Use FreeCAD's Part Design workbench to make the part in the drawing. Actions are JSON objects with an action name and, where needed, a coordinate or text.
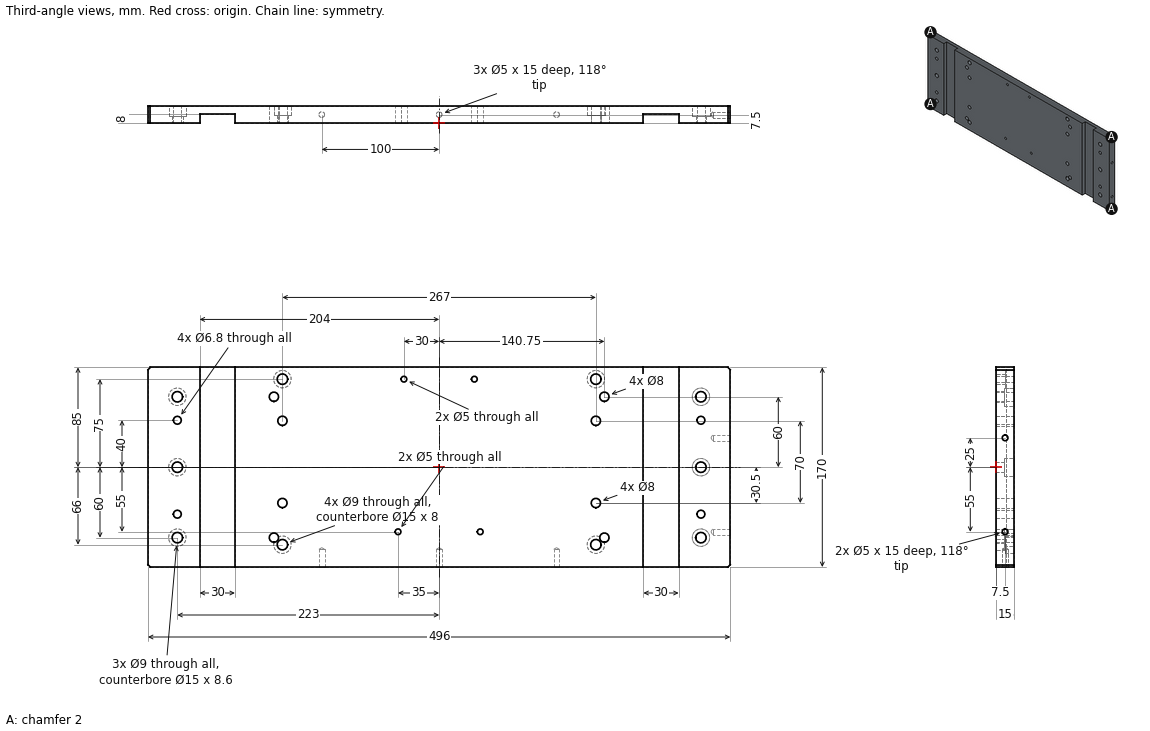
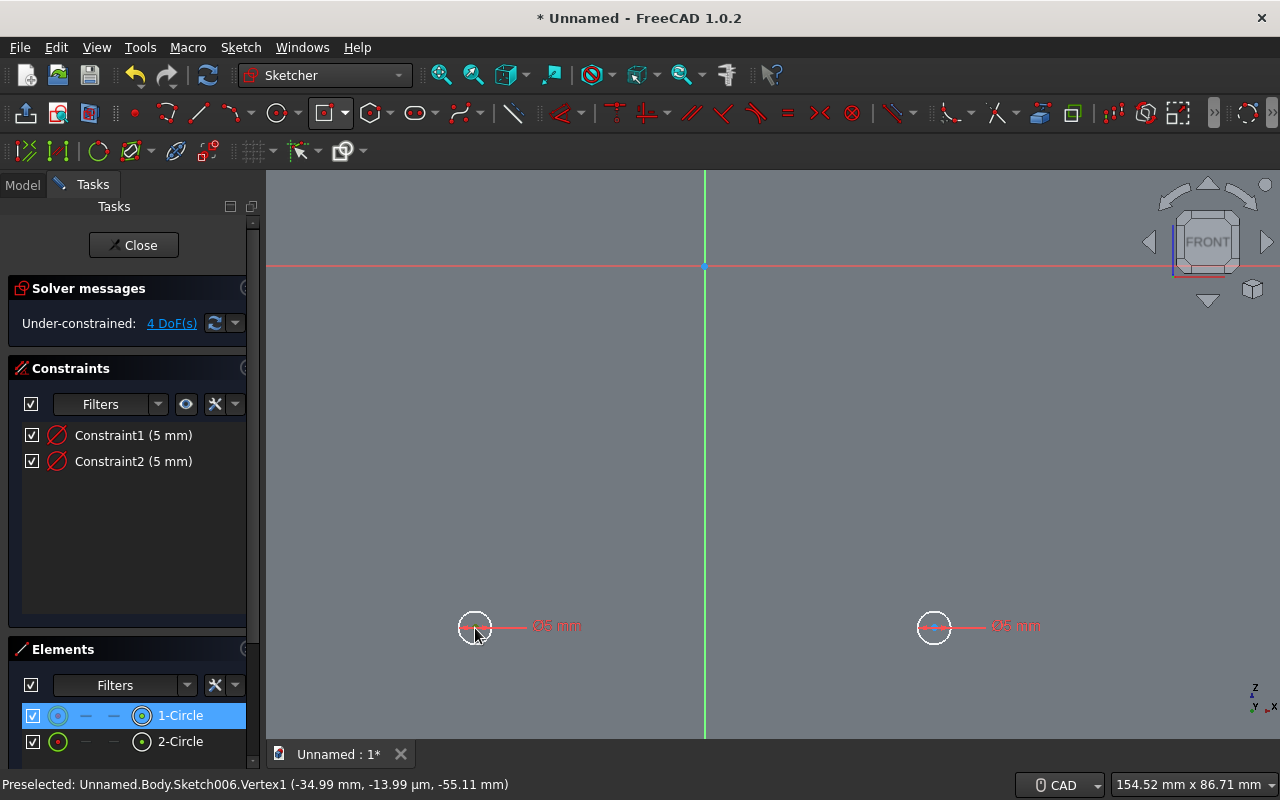
{"action": "left_click", "coordinate": [934, 628]}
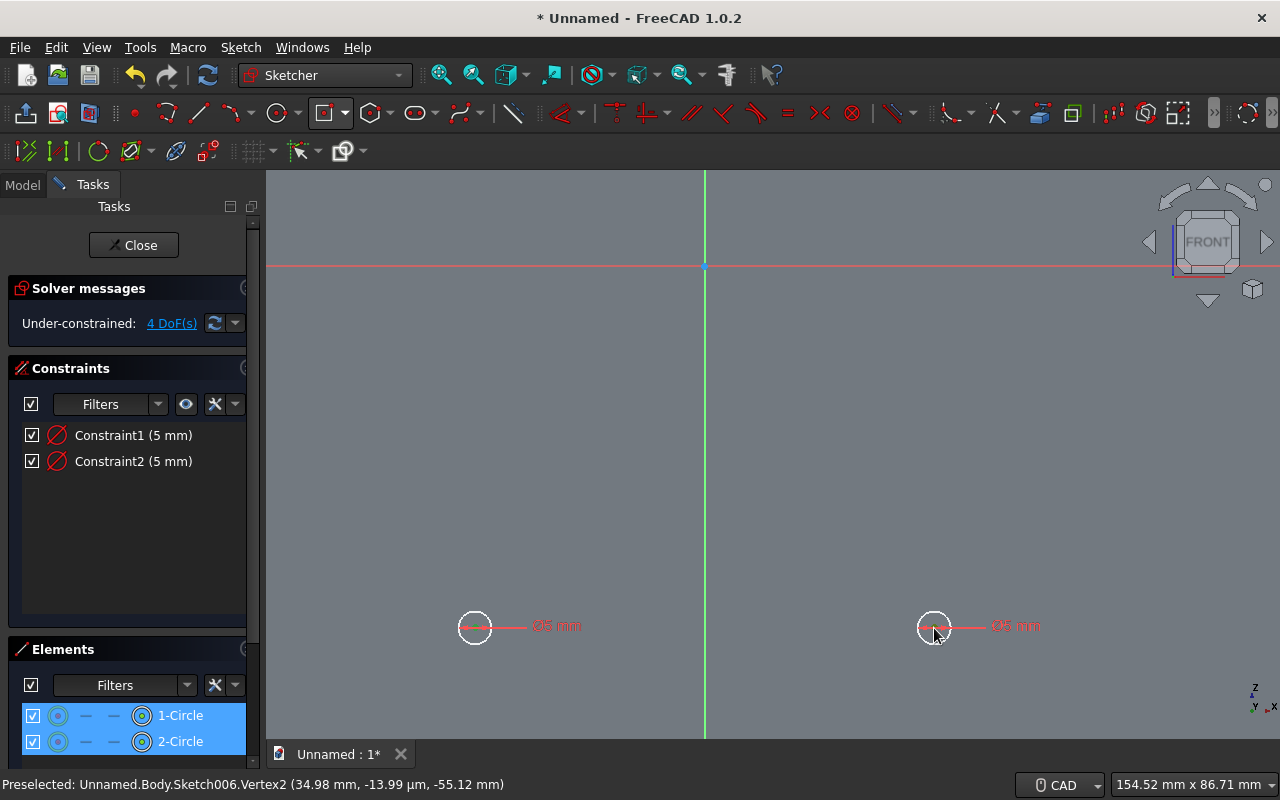
{"action": "left_click", "coordinate": [705, 674]}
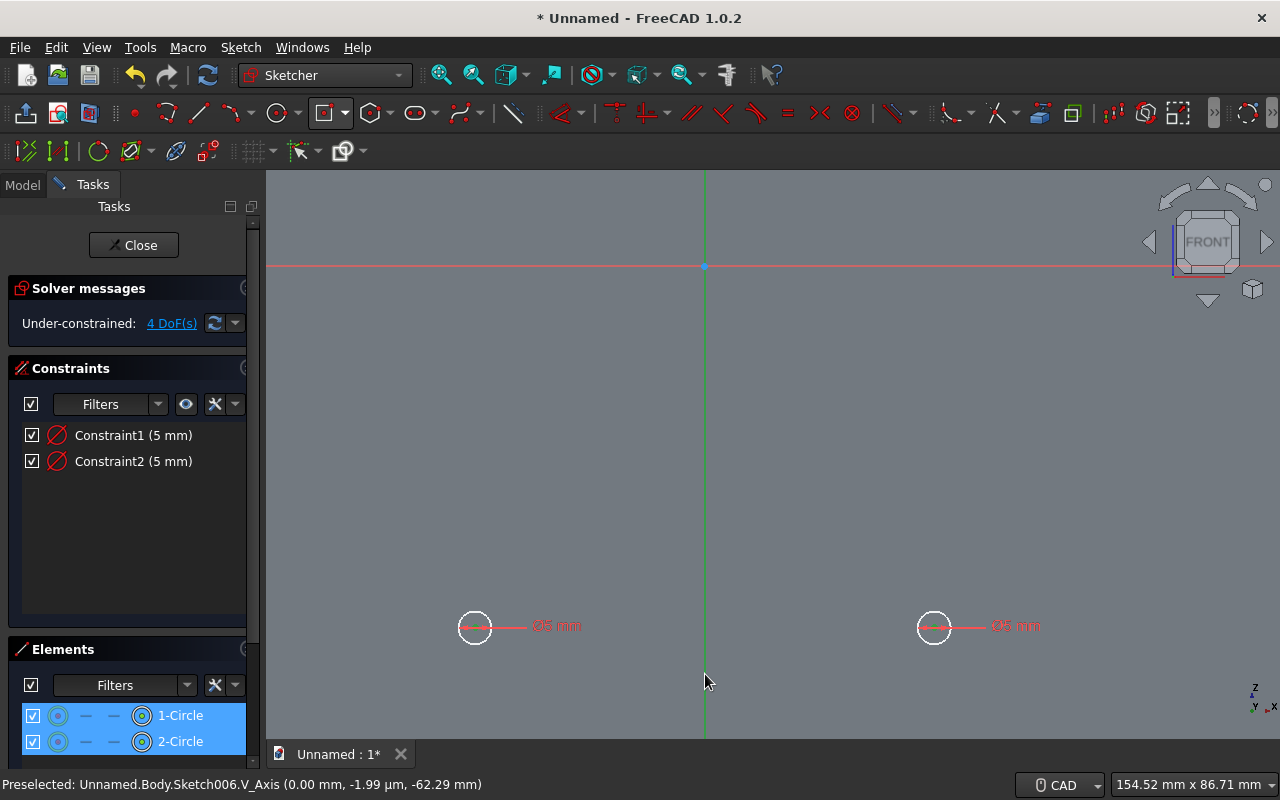
{"action": "left_click", "coordinate": [820, 114]}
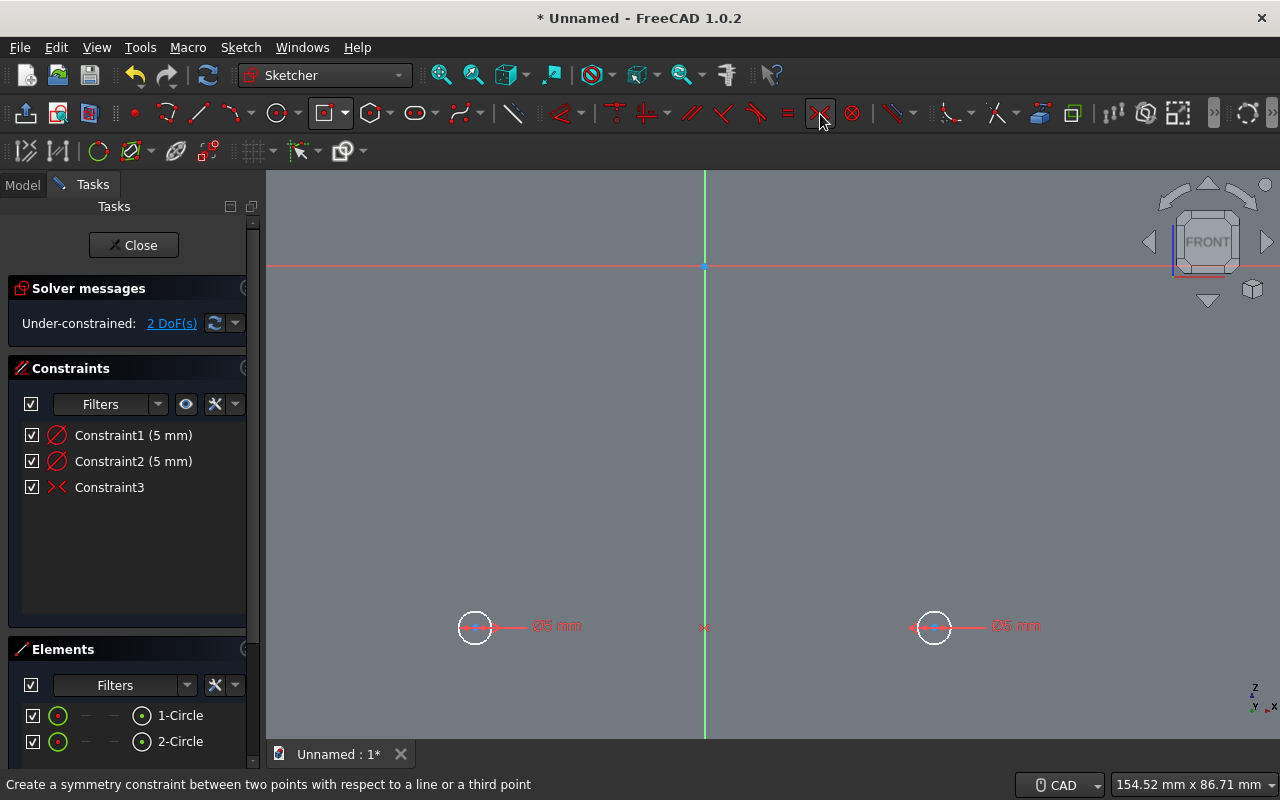
{"action": "left_click", "coordinate": [560, 114]}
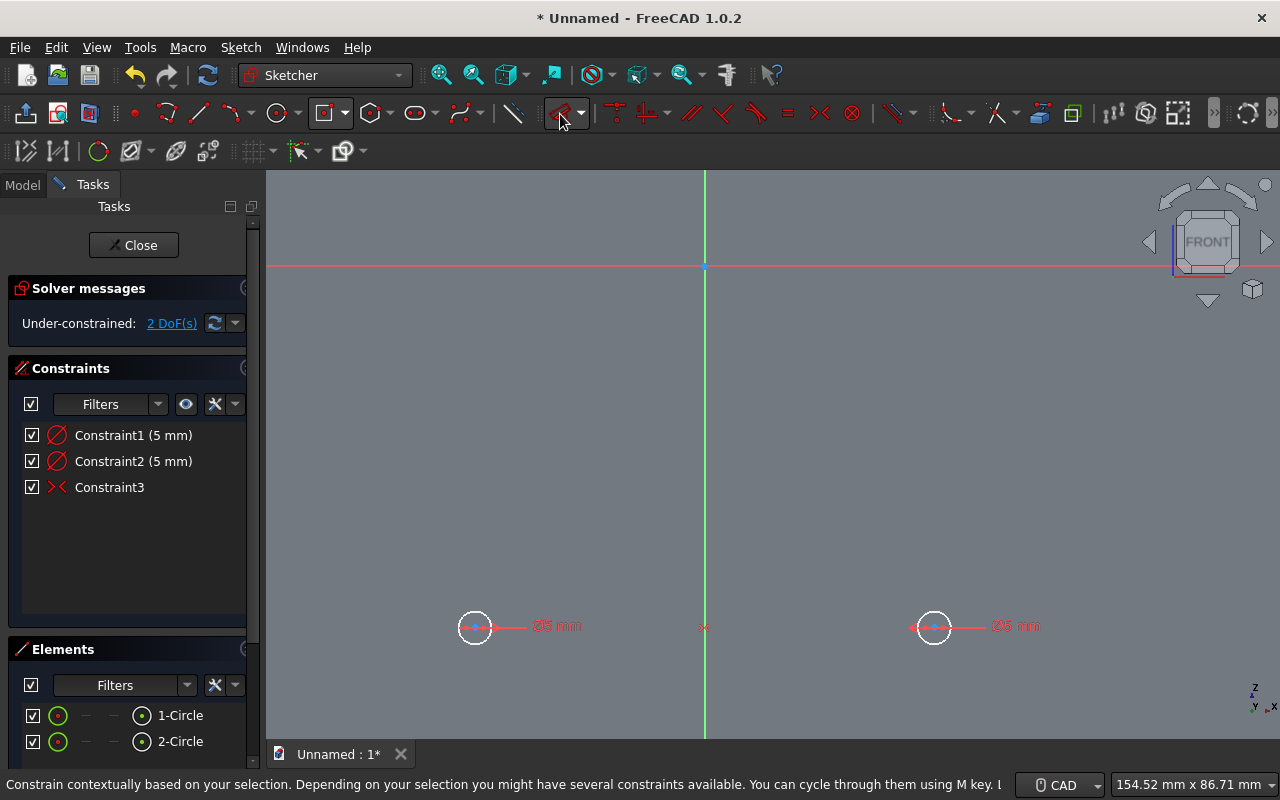
{"action": "left_click", "coordinate": [475, 628]}
{"action": "left_click", "coordinate": [590, 232]}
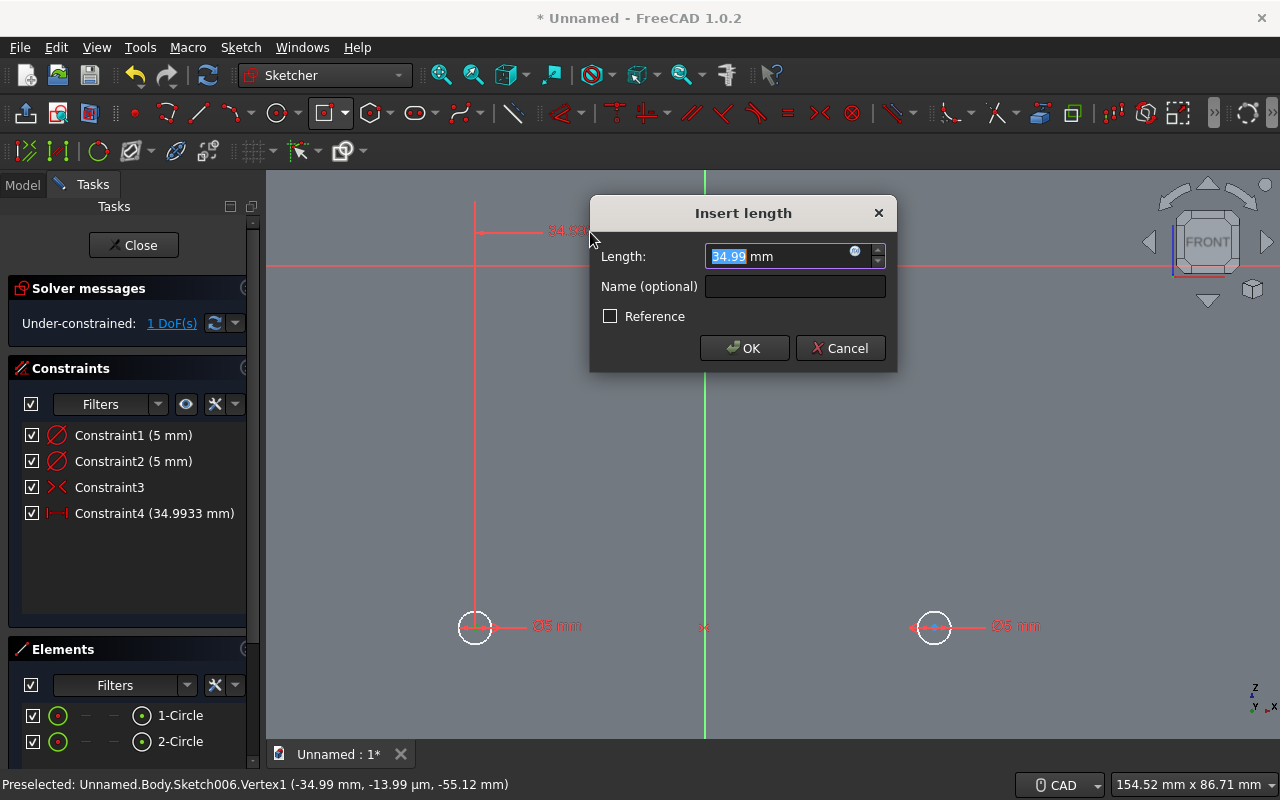
{"action": "type", "text": "35"}
{"action": "key", "text": "Return"}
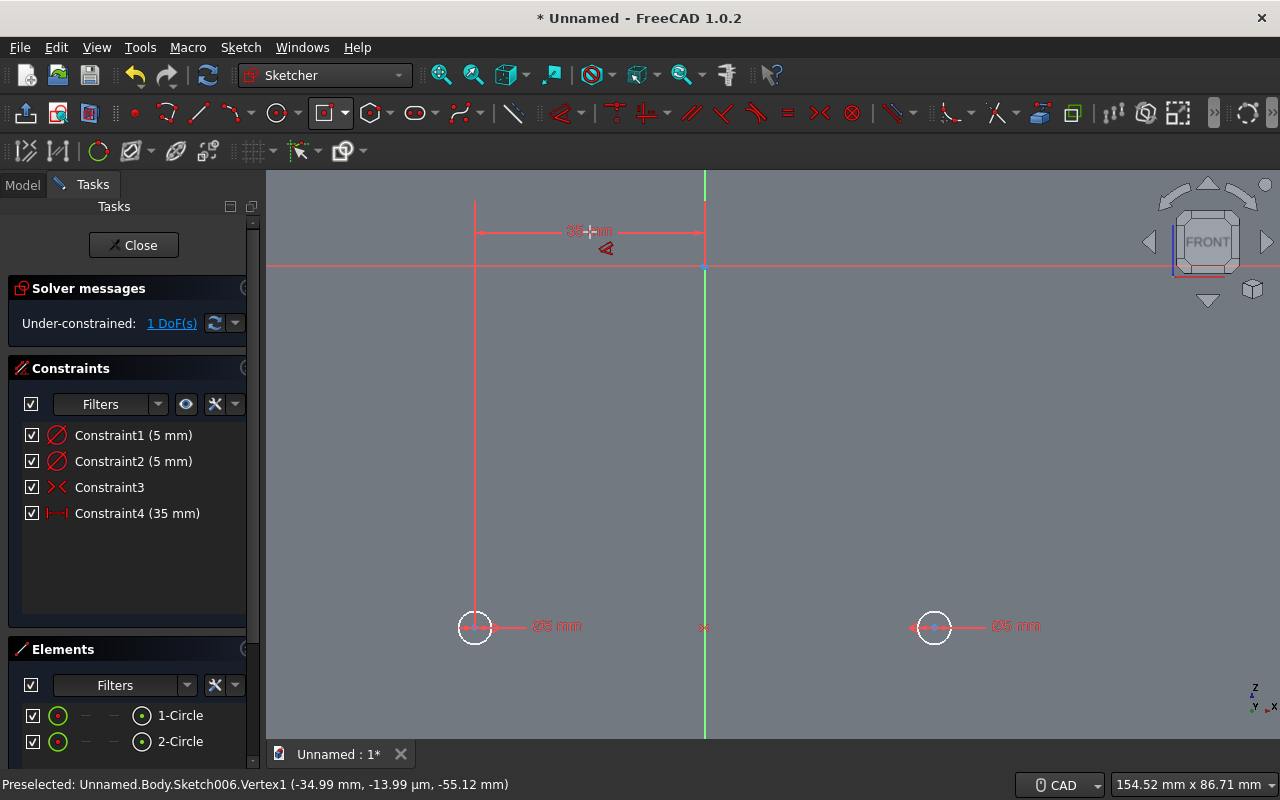
{"action": "left_click", "coordinate": [475, 628]}
{"action": "left_click", "coordinate": [441, 447]}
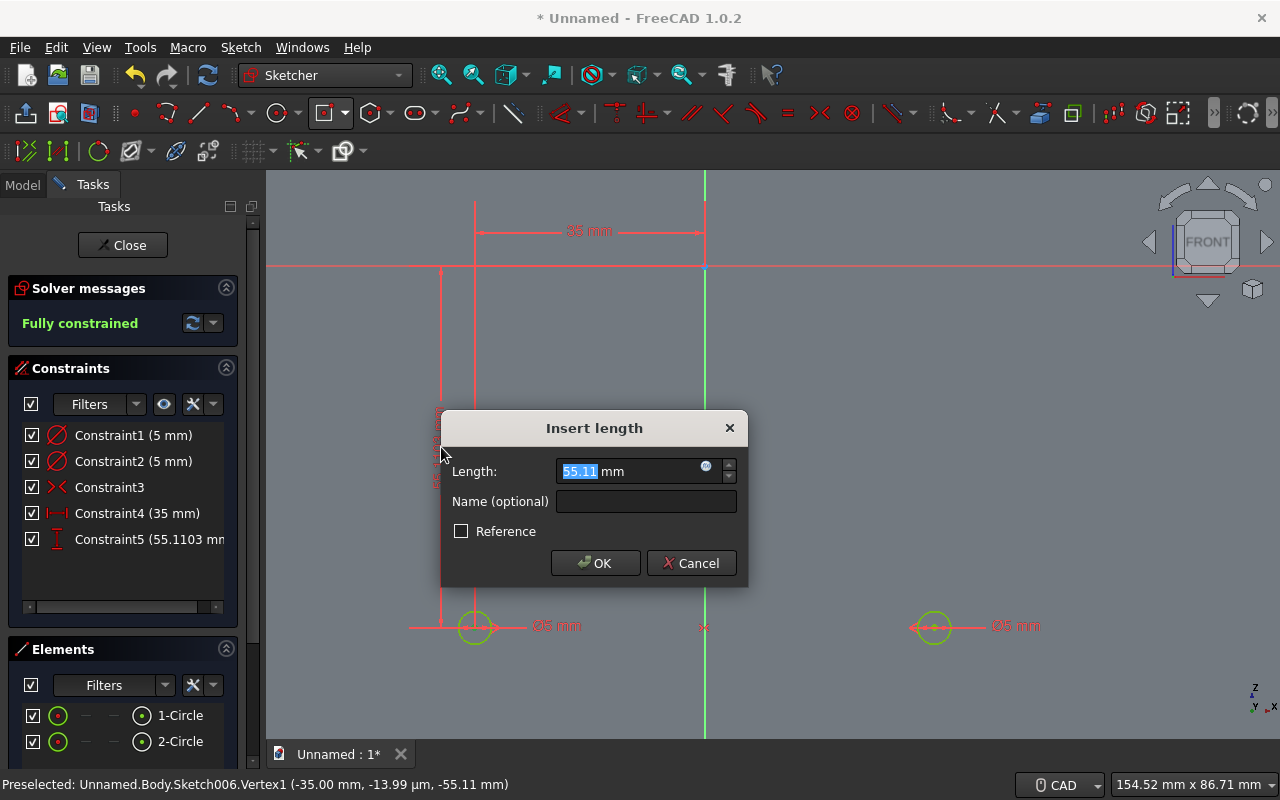
{"action": "type", "text": "55"}
{"action": "key", "text": "Return"}
{"action": "key", "text": "Escape"}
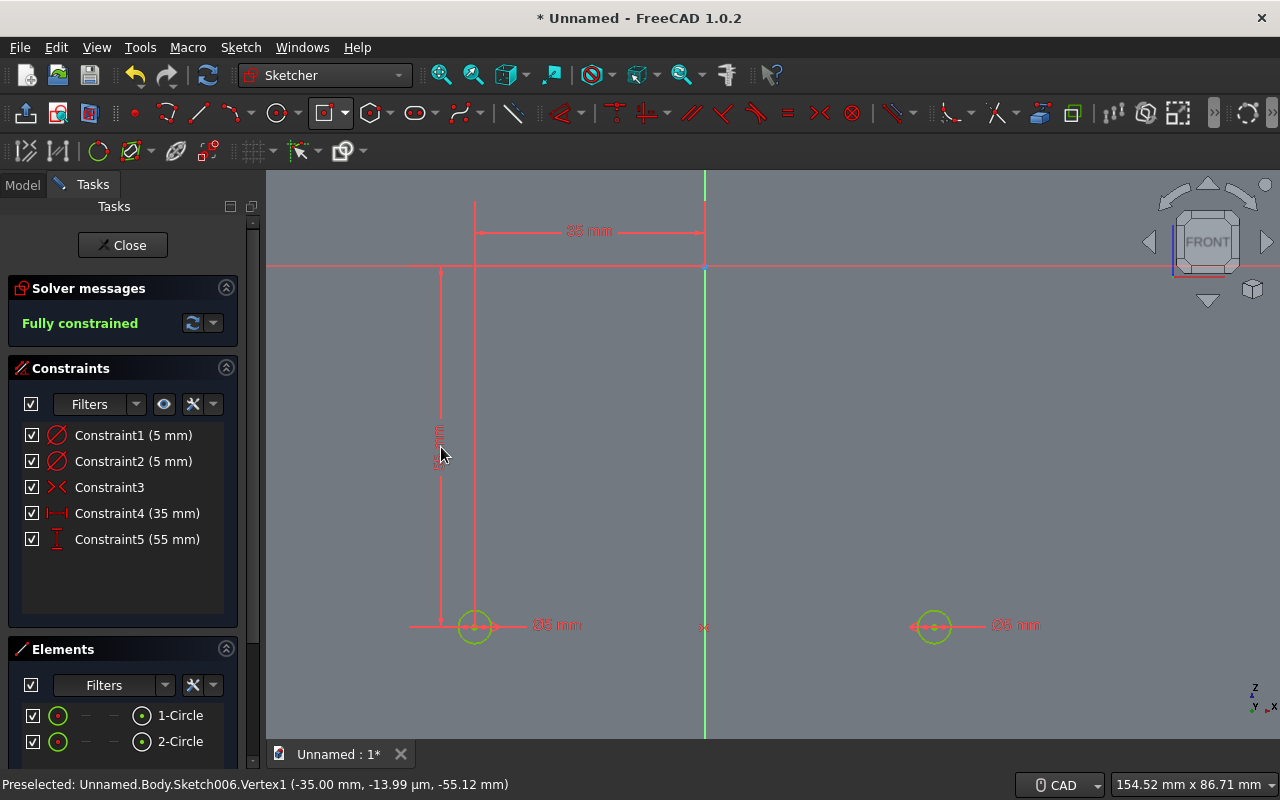
{"action": "left_click", "coordinate": [123, 245]}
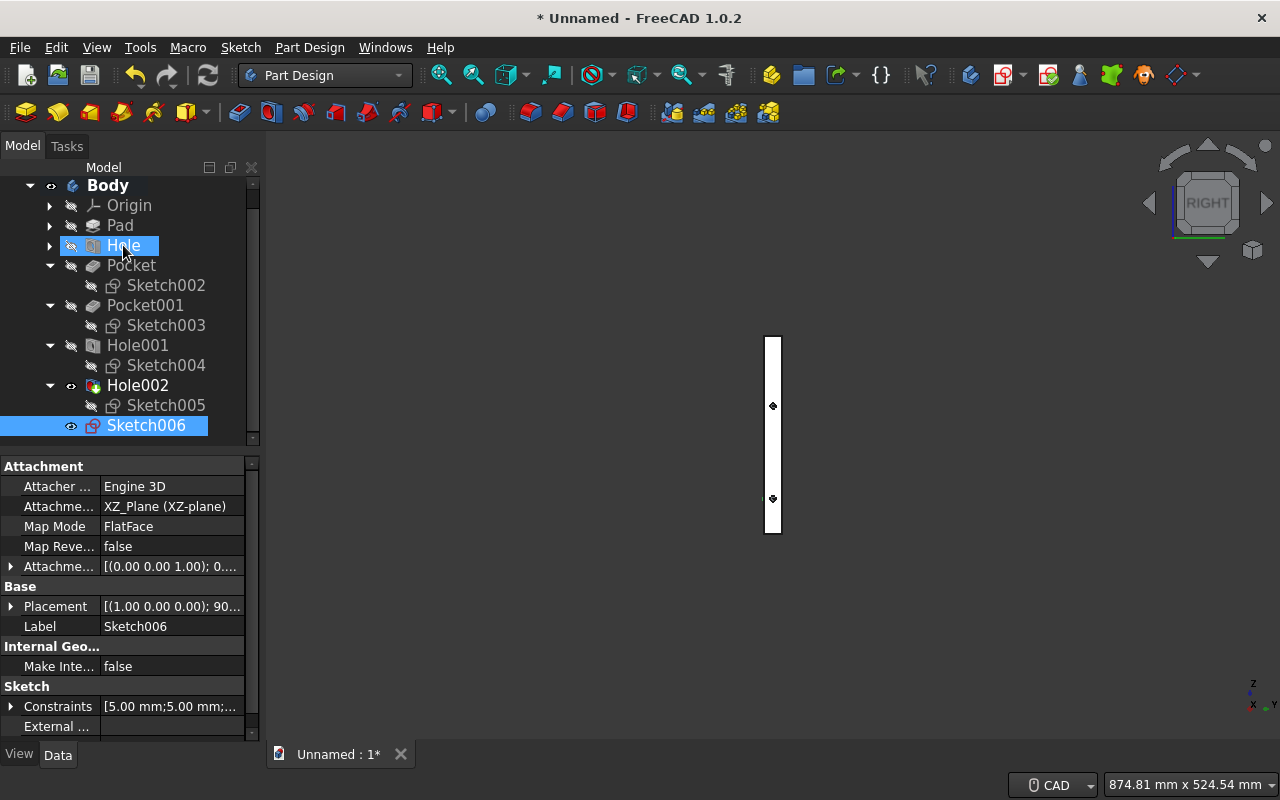
{"action": "left_click", "coordinate": [272, 112]}